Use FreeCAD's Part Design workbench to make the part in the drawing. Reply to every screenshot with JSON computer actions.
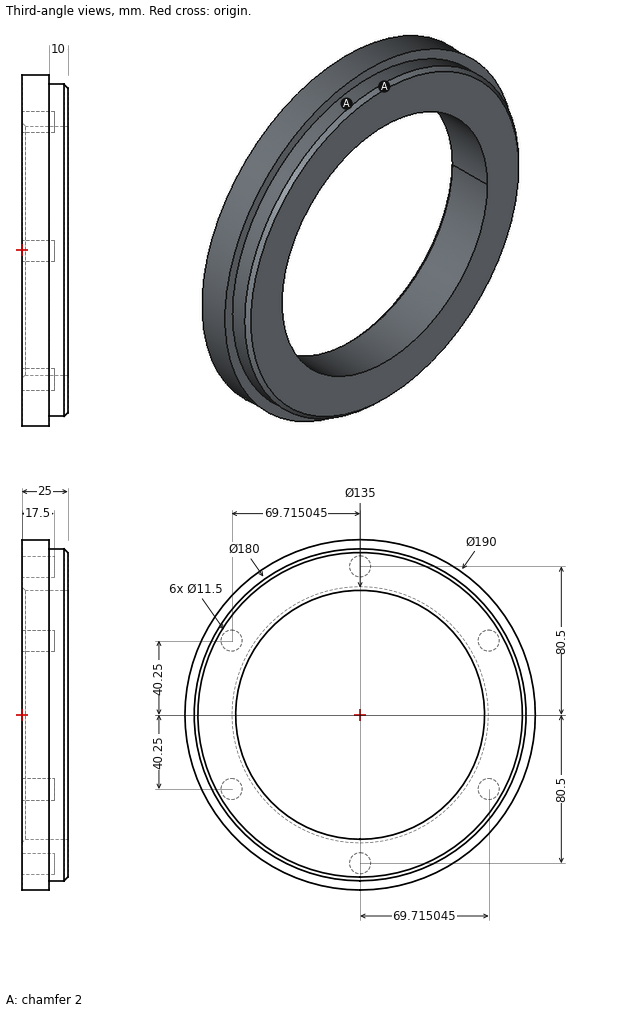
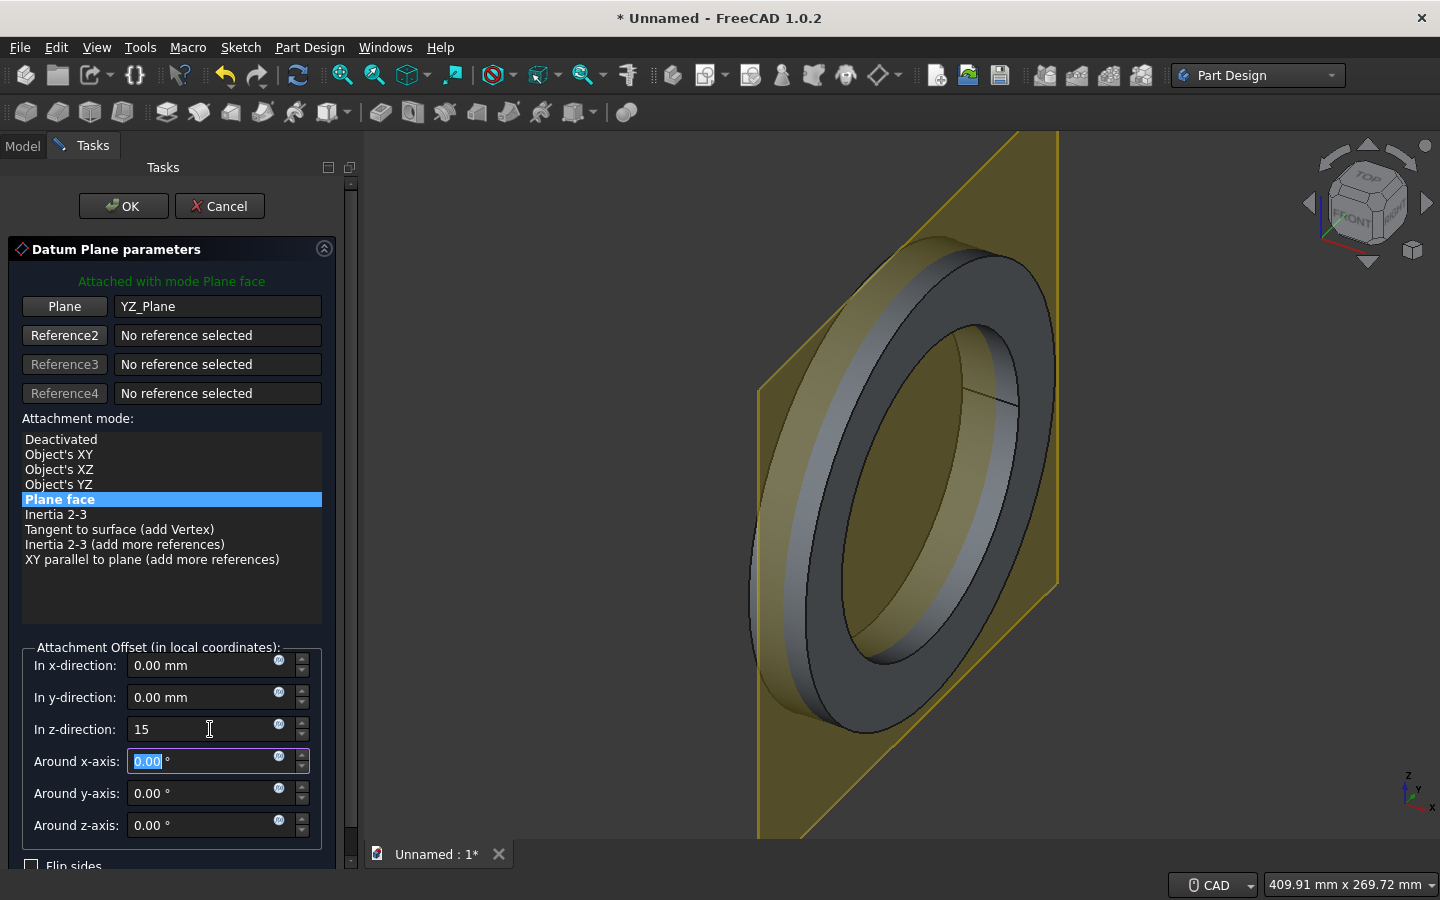
{"action": "left_click", "coordinate": [124, 206]}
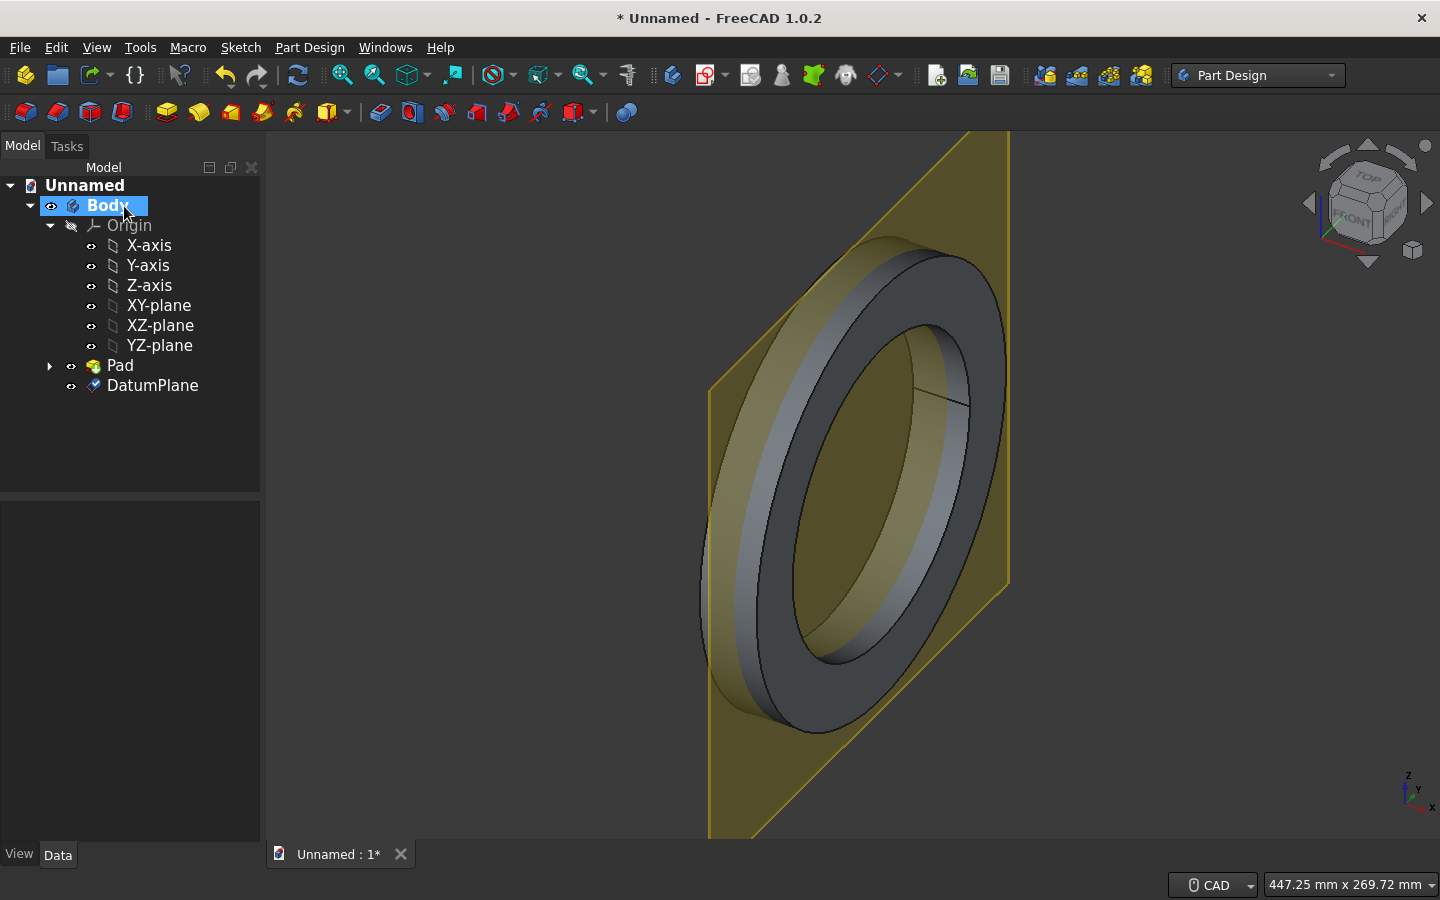
{"action": "left_click", "coordinate": [116, 386]}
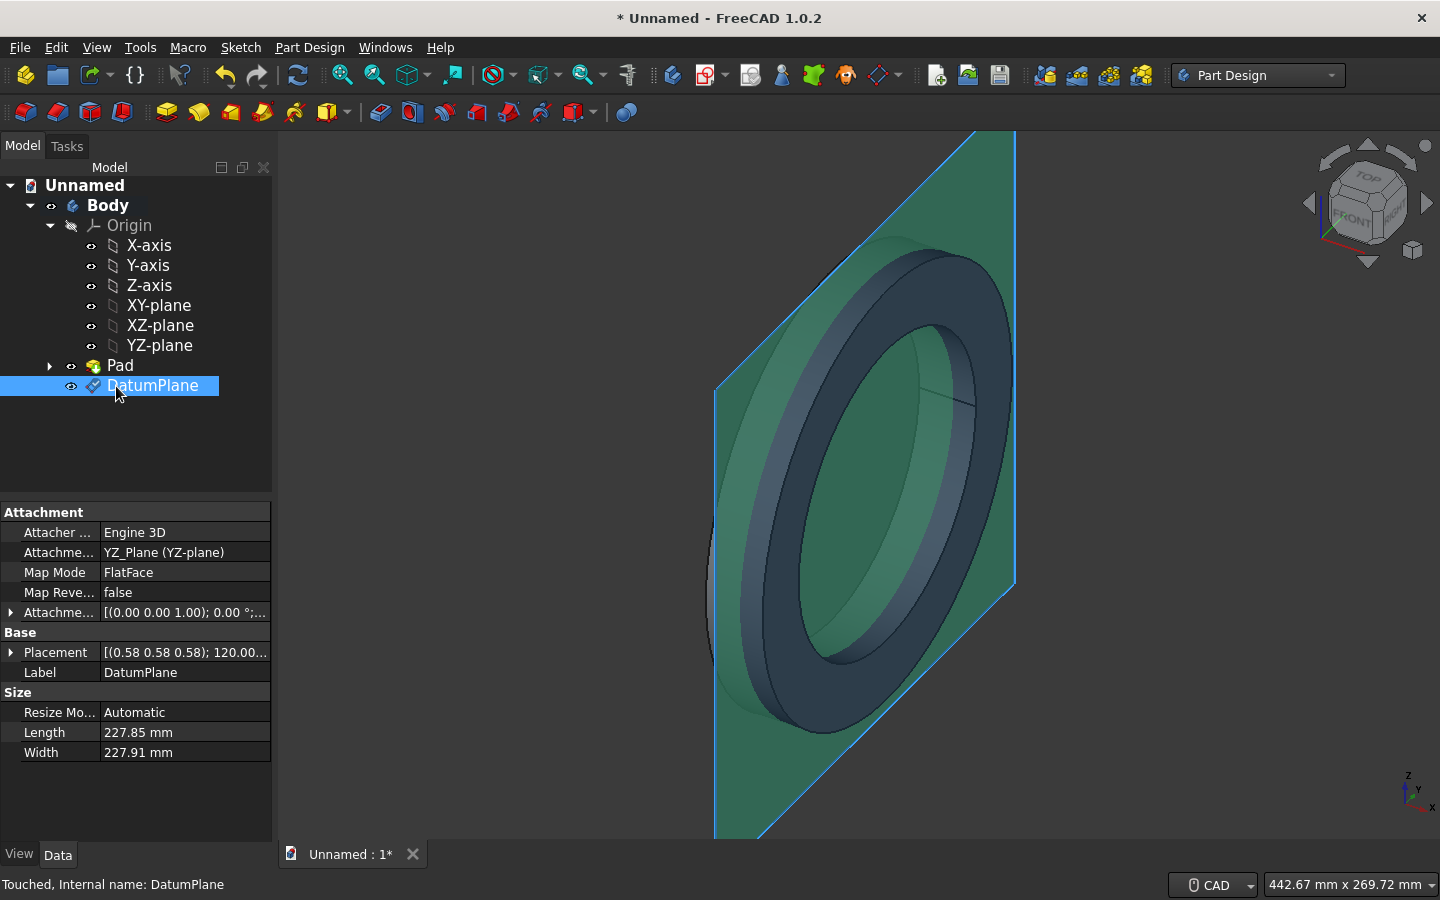
{"action": "left_click", "coordinate": [706, 76]}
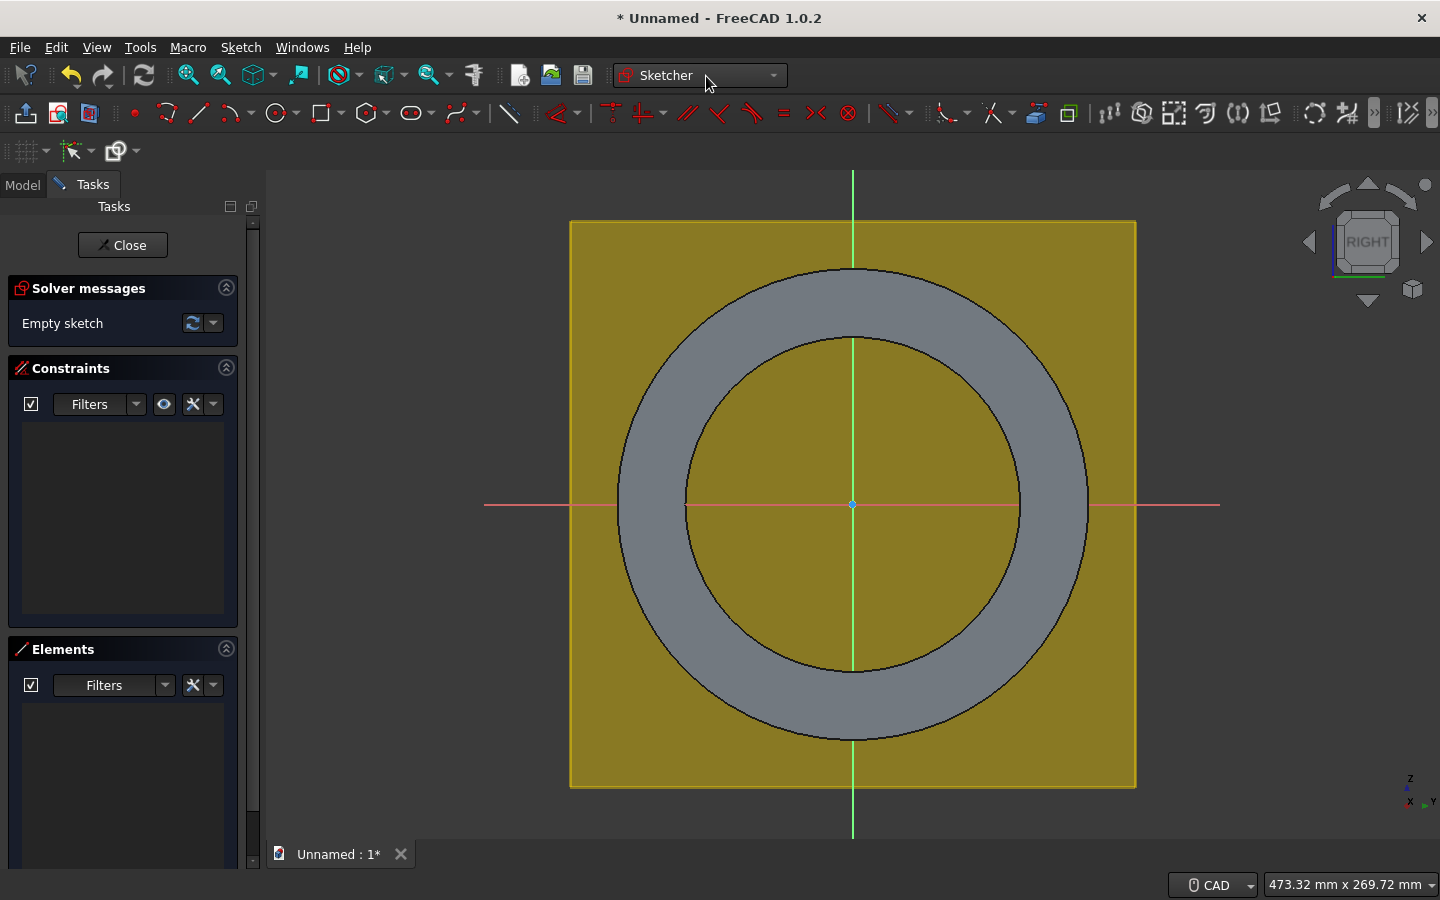
{"action": "left_click", "coordinate": [90, 114]}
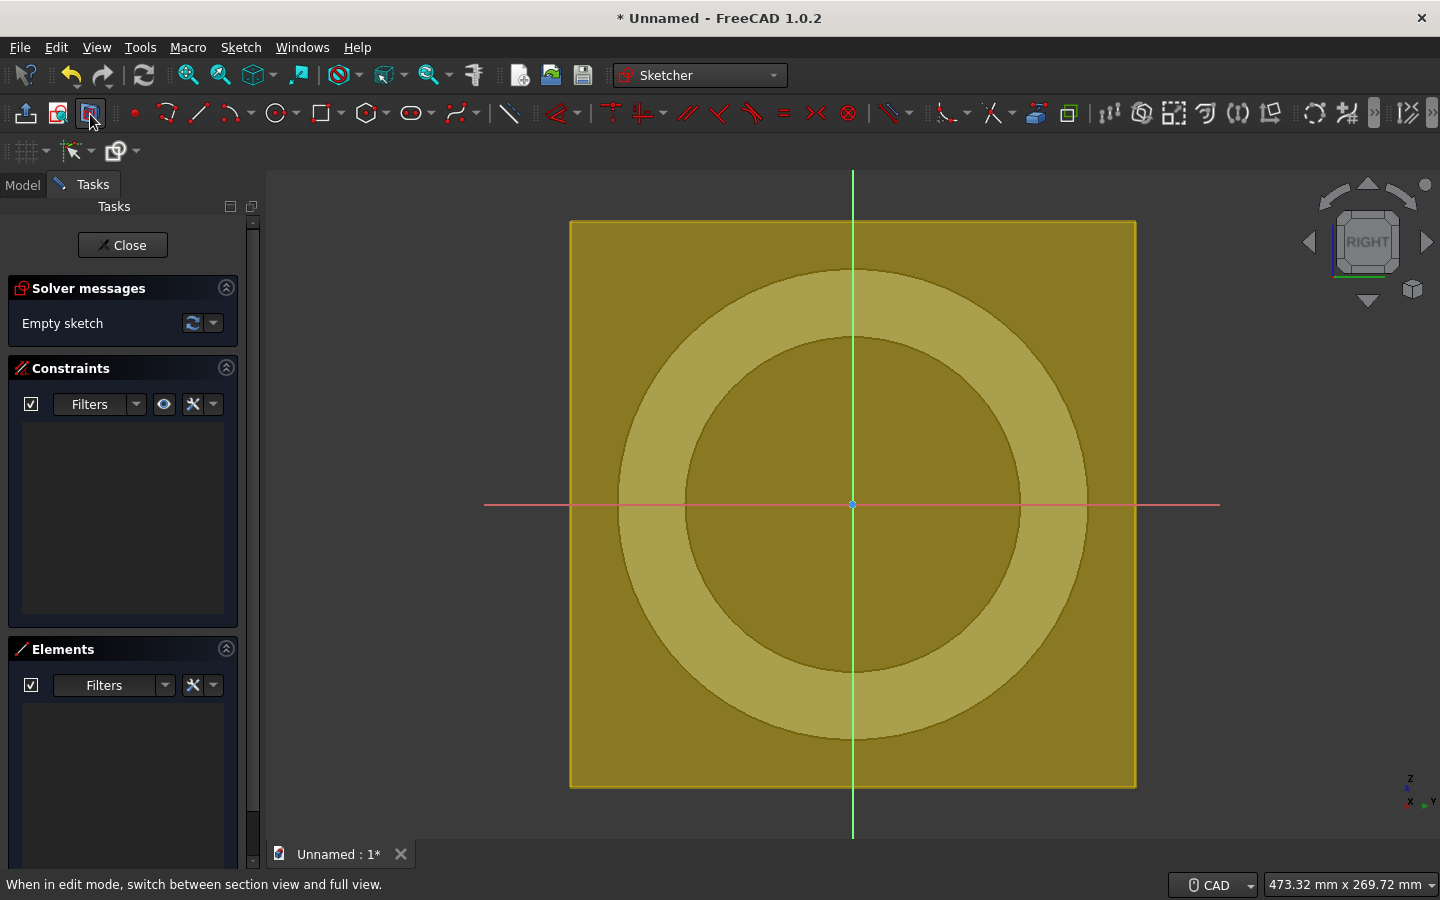
{"action": "left_click", "coordinate": [276, 114]}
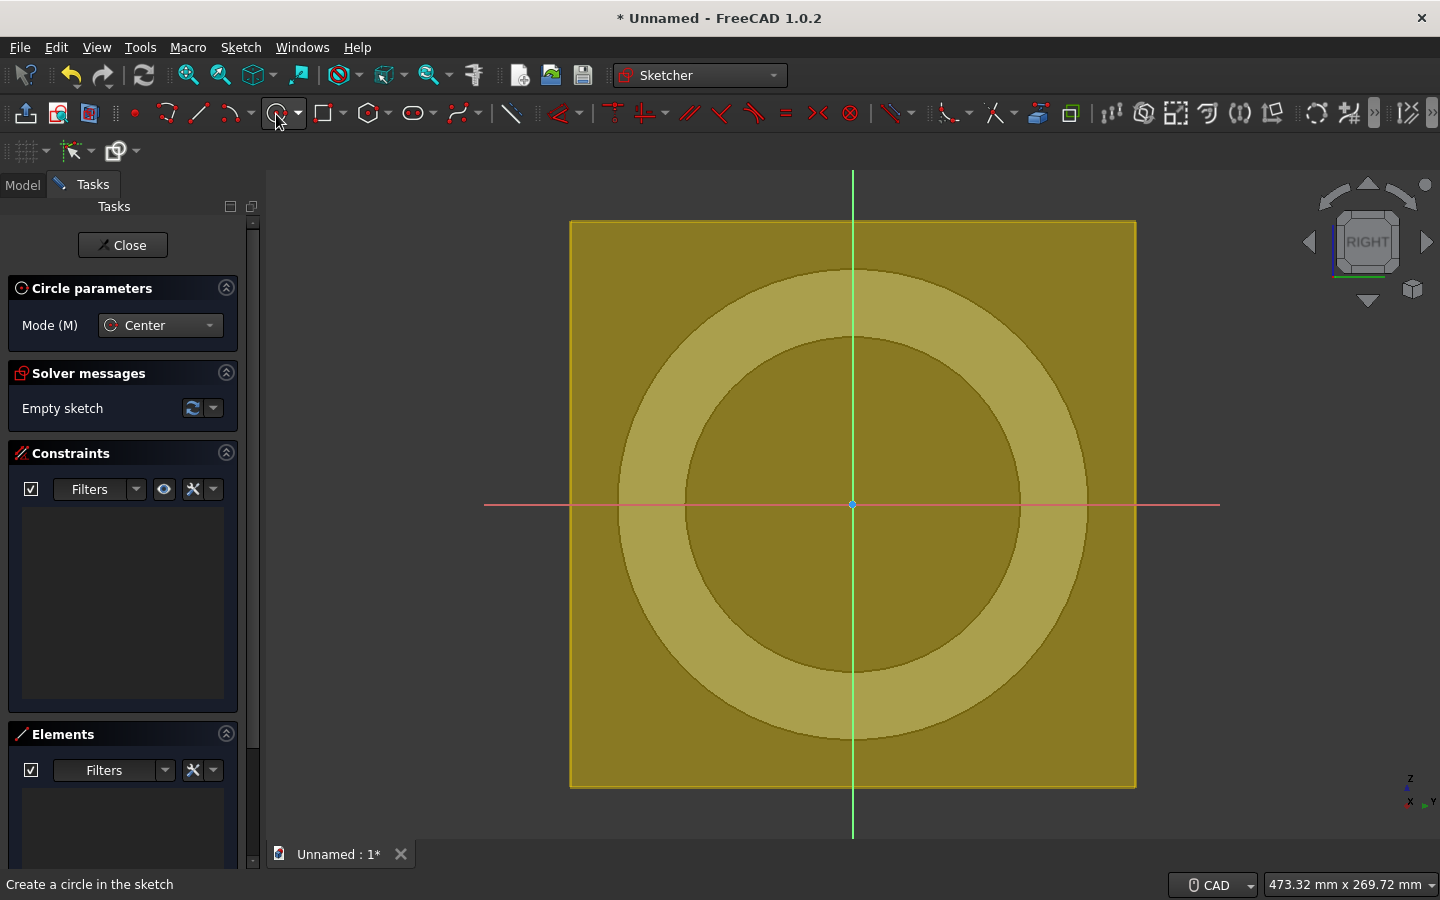
{"action": "left_click", "coordinate": [853, 504]}
{"action": "left_click", "coordinate": [1019, 338]}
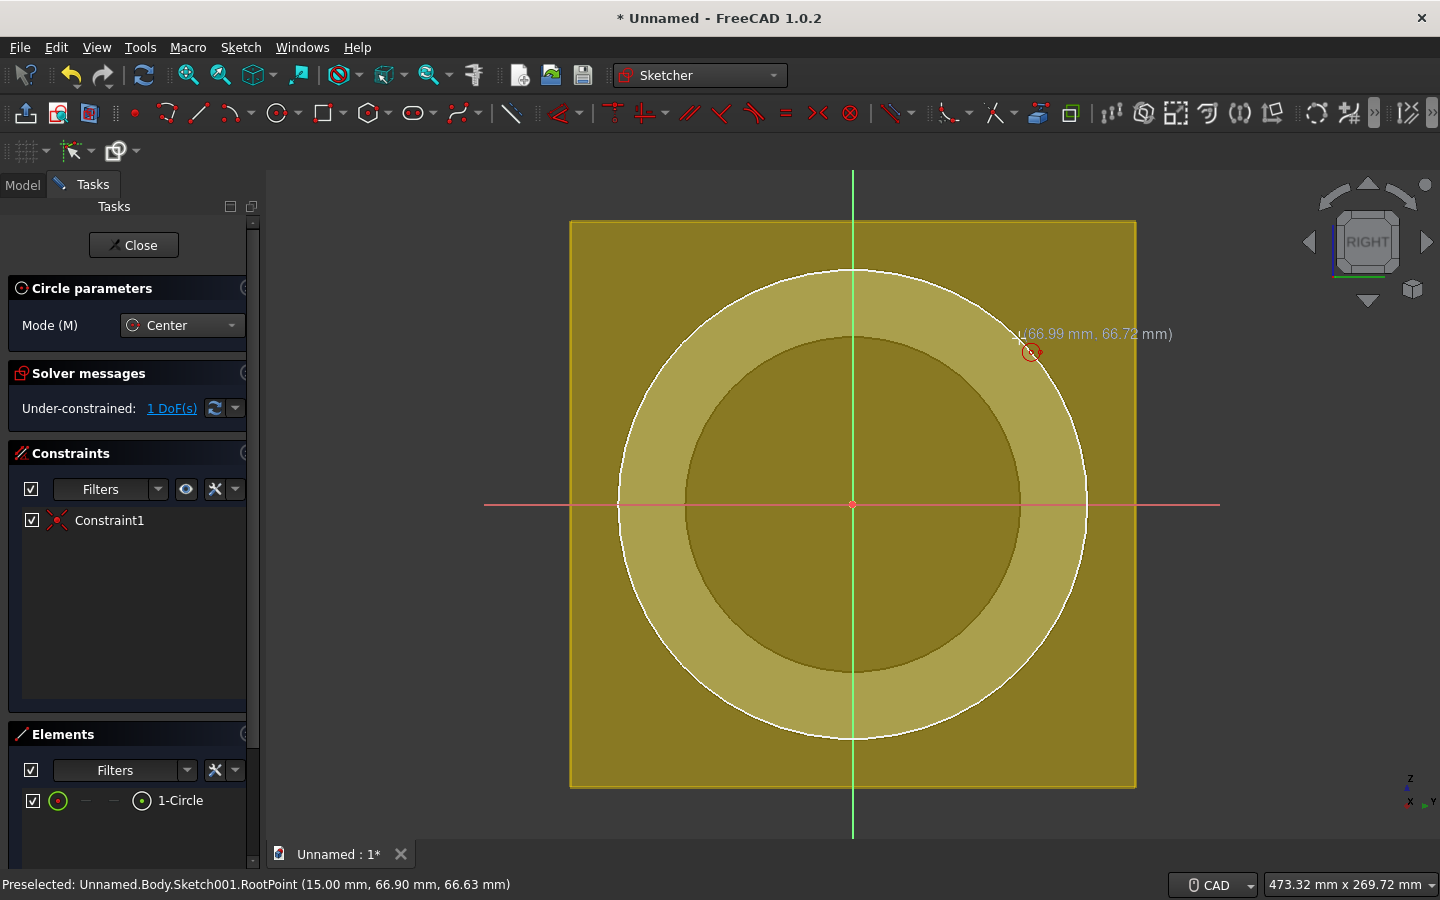
{"action": "left_click", "coordinate": [853, 504]}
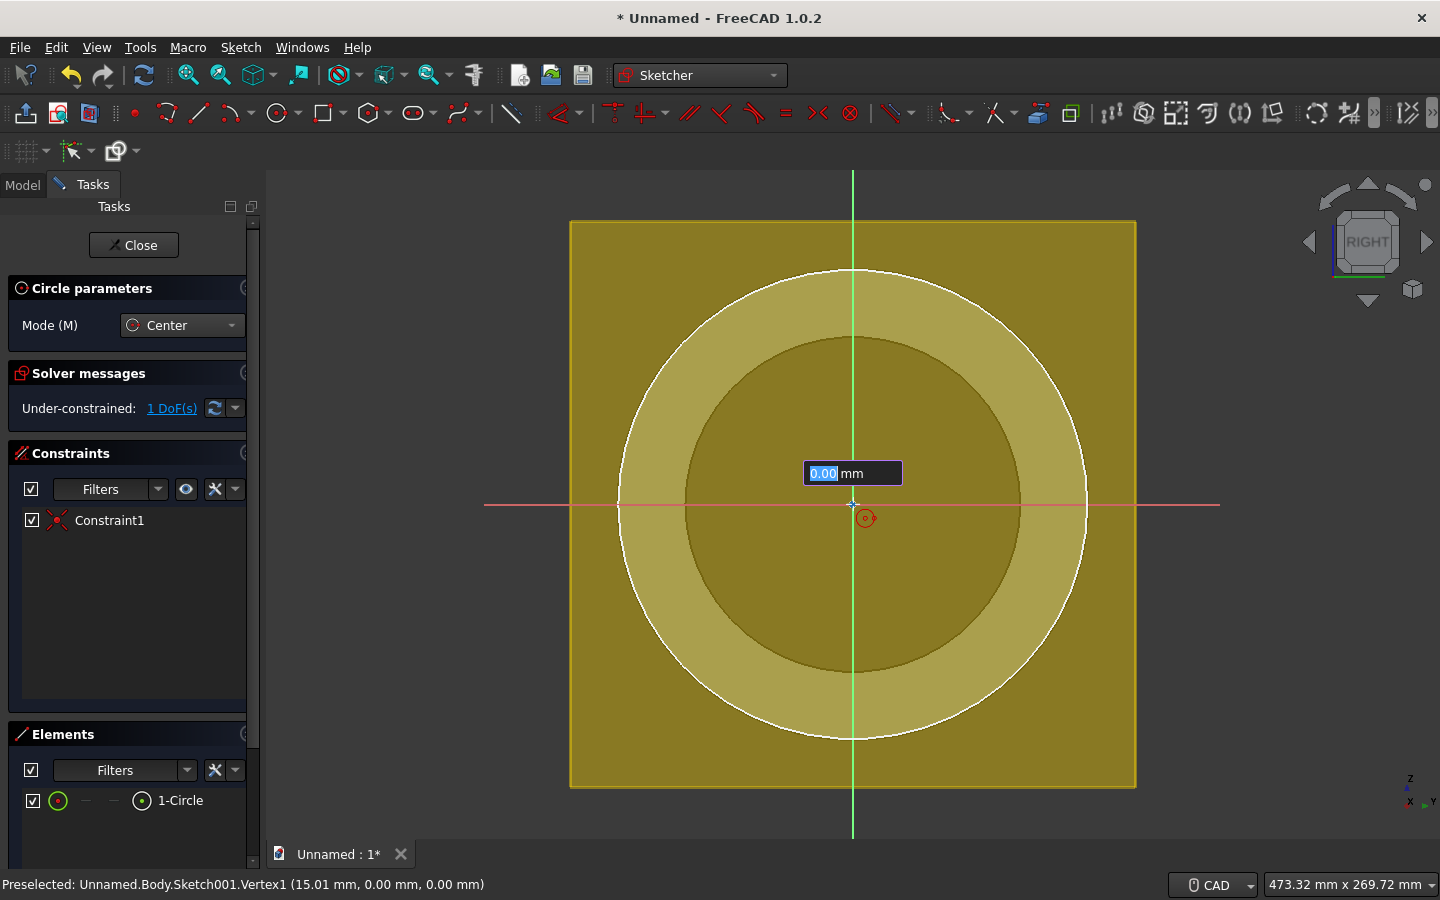
{"action": "scroll", "coordinate": [1011, 347], "scroll_direction": "up", "scroll_amount": 2}